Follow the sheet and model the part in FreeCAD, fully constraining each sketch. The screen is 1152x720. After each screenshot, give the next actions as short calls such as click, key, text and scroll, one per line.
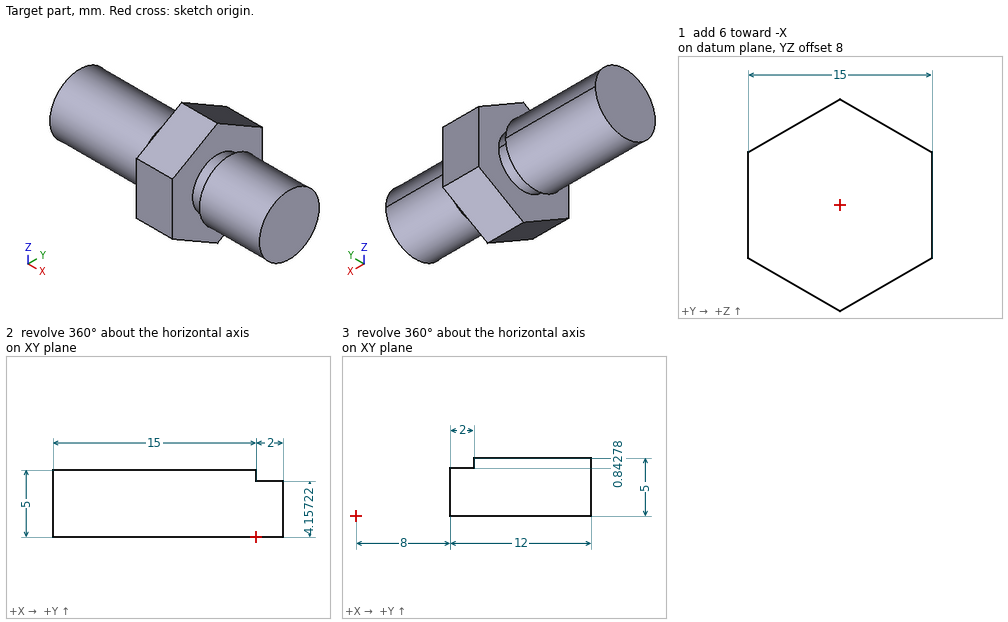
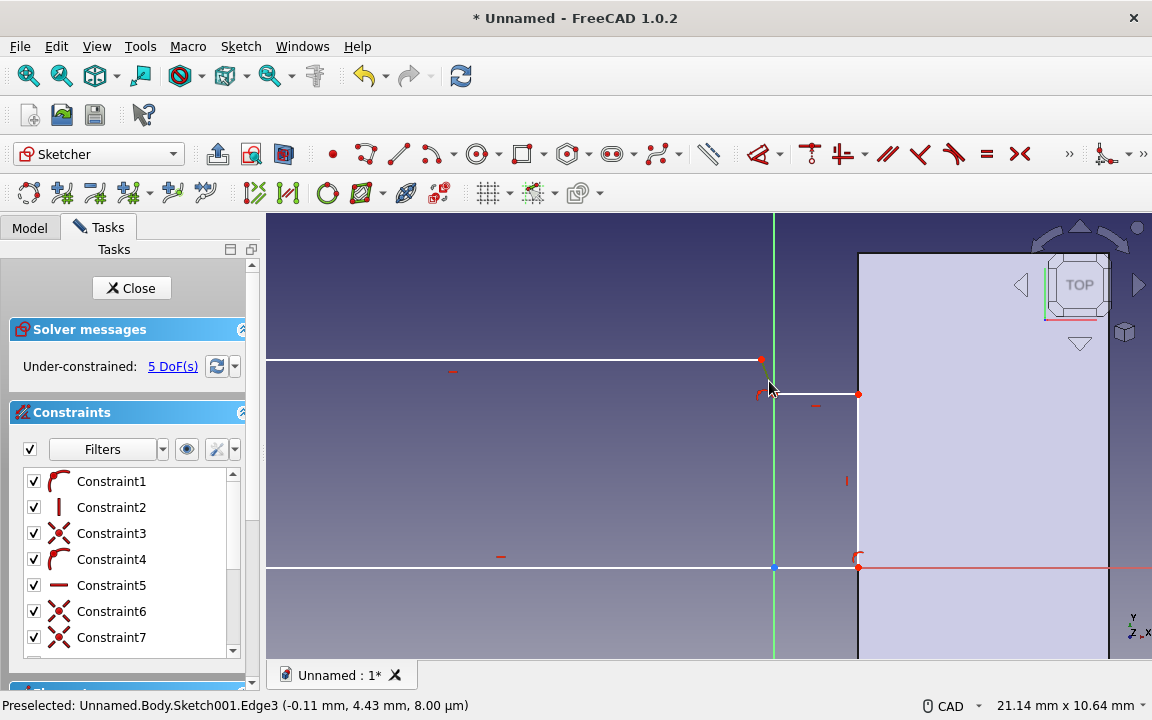
key(v)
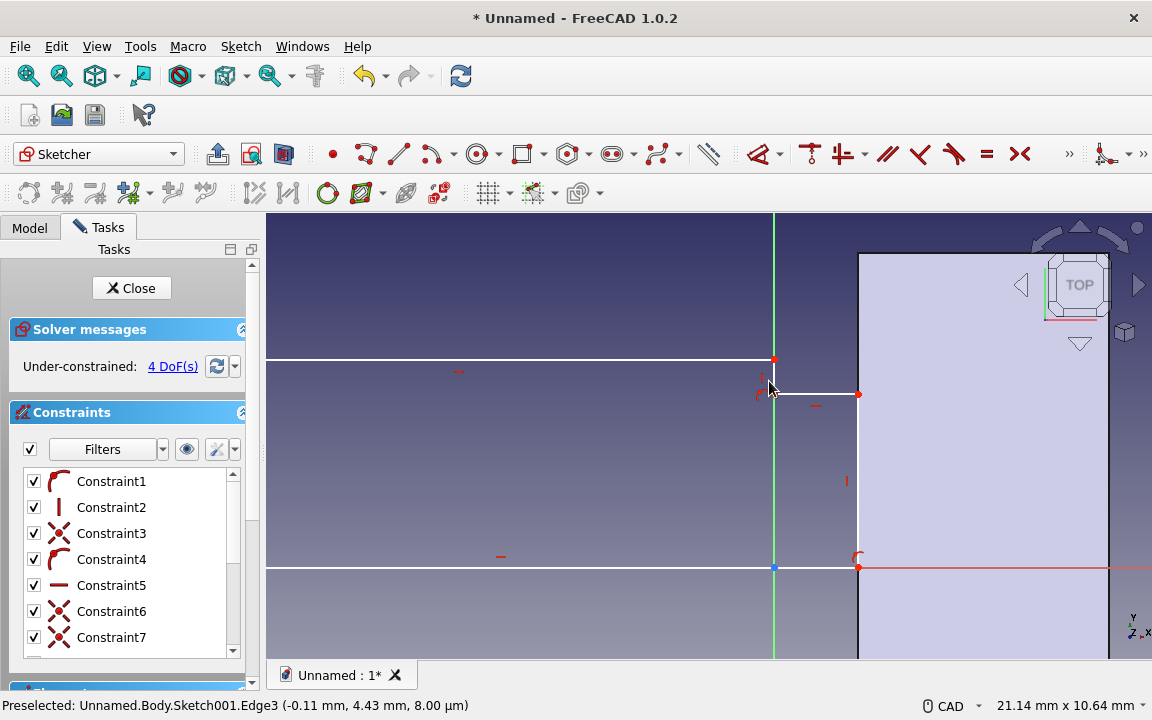
click(833, 394)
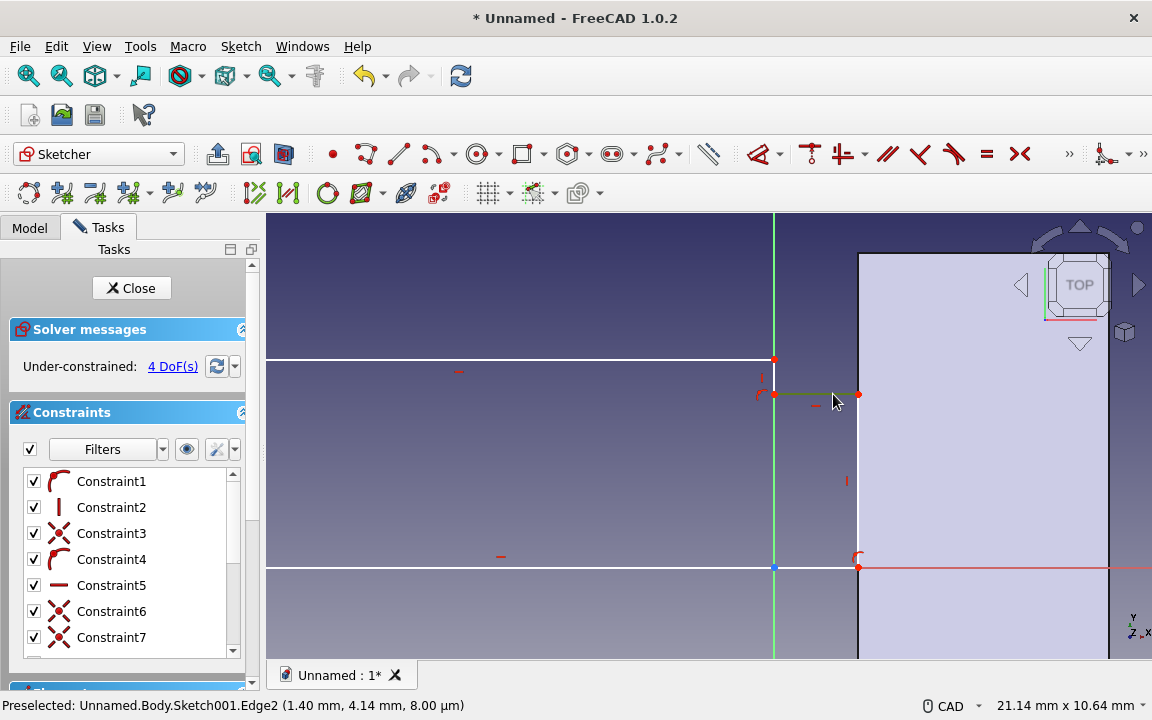
key(l)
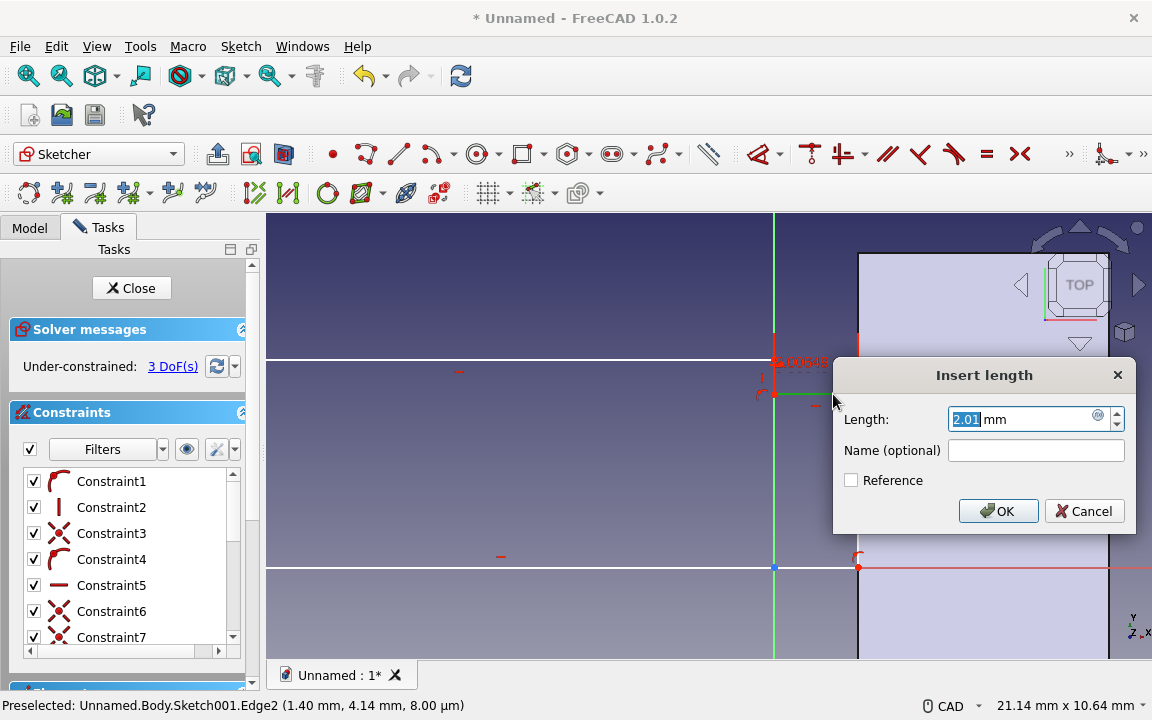
text(2)
key(Return)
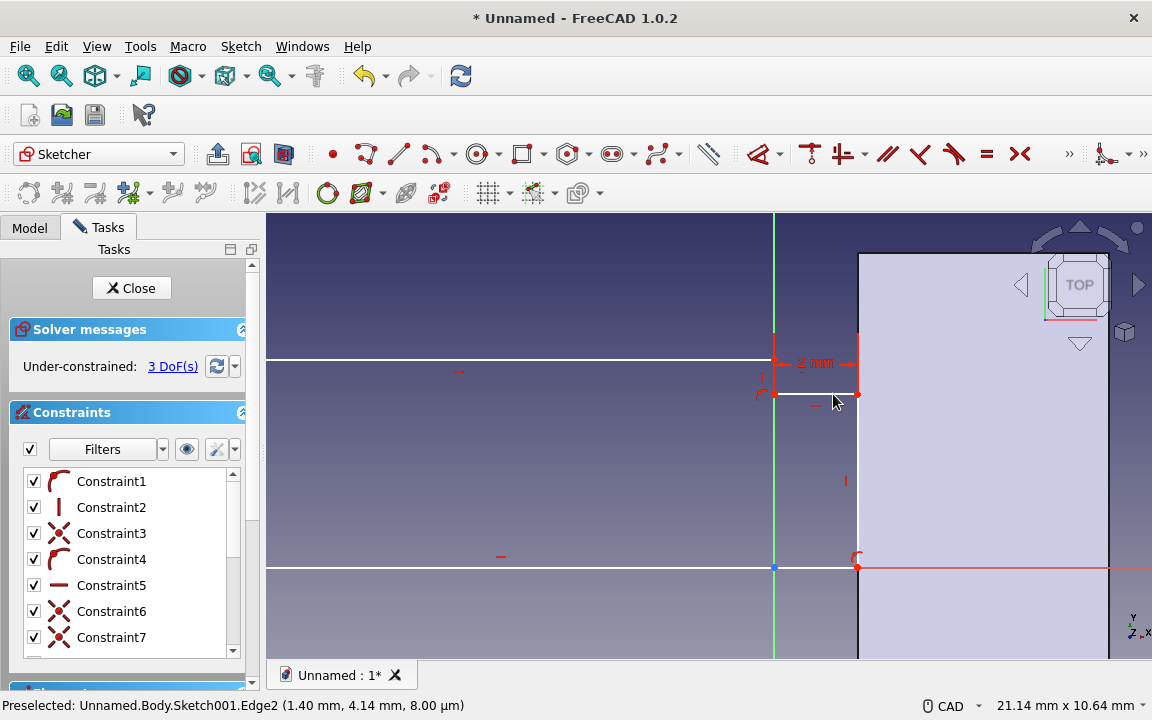
scroll(923, 381, down, 2)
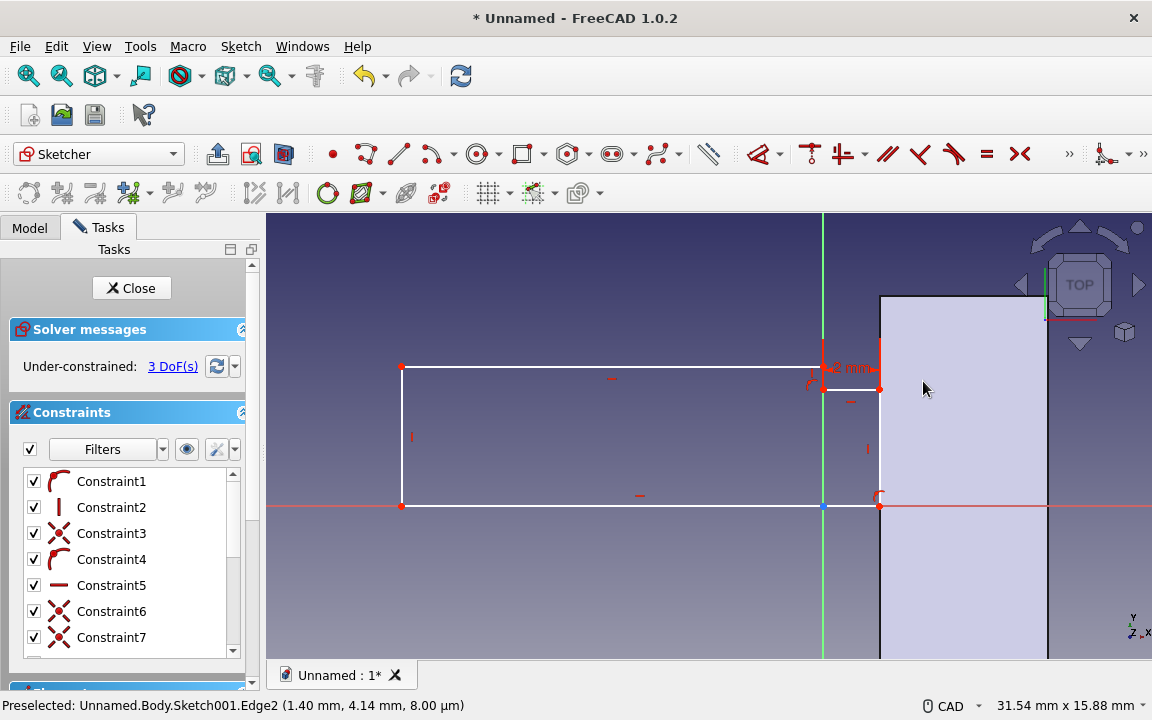
click(402, 409)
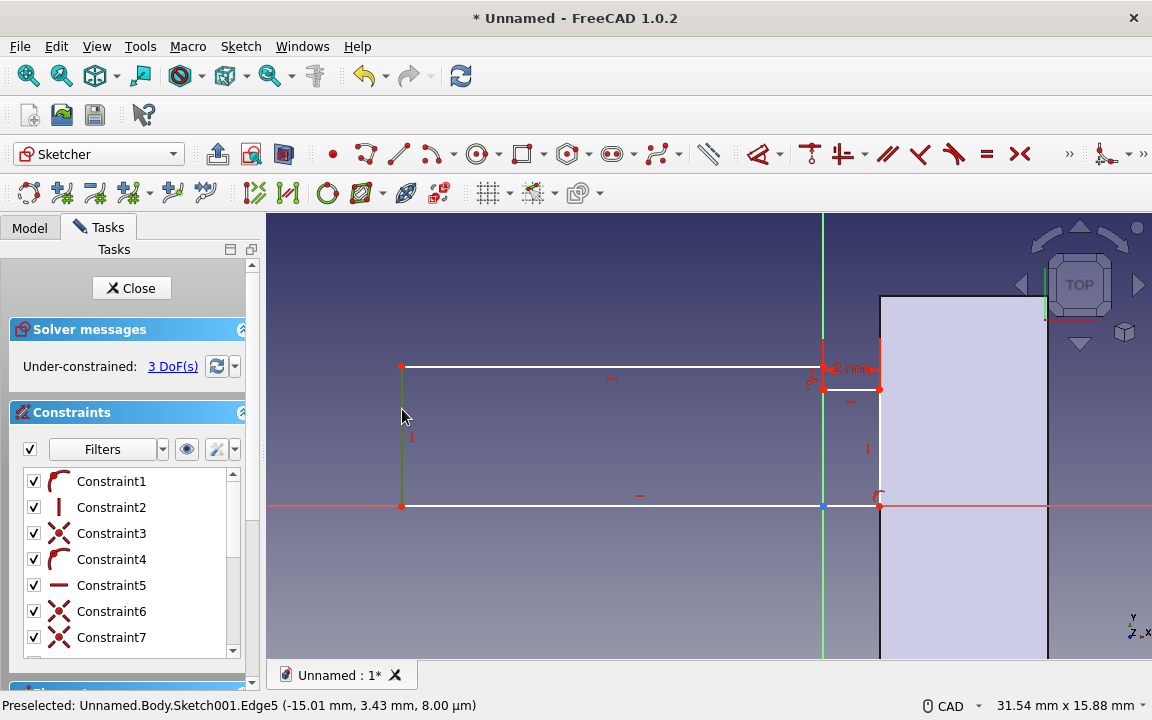
key(i)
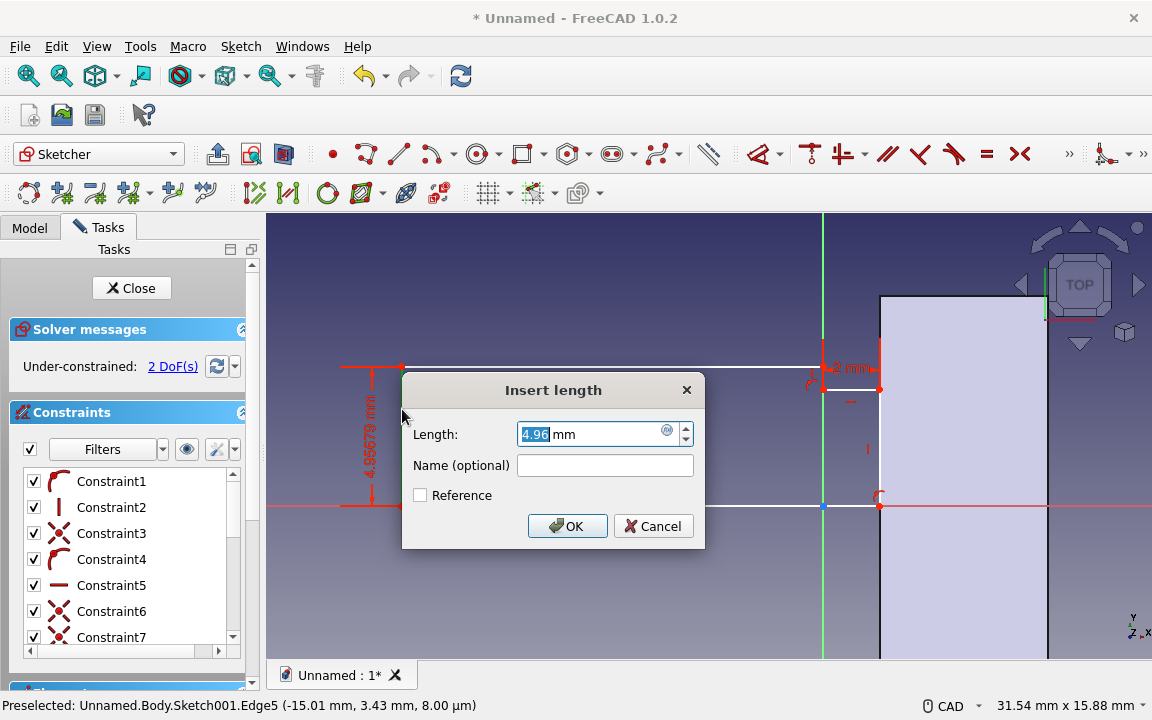
text(5)
key(Return)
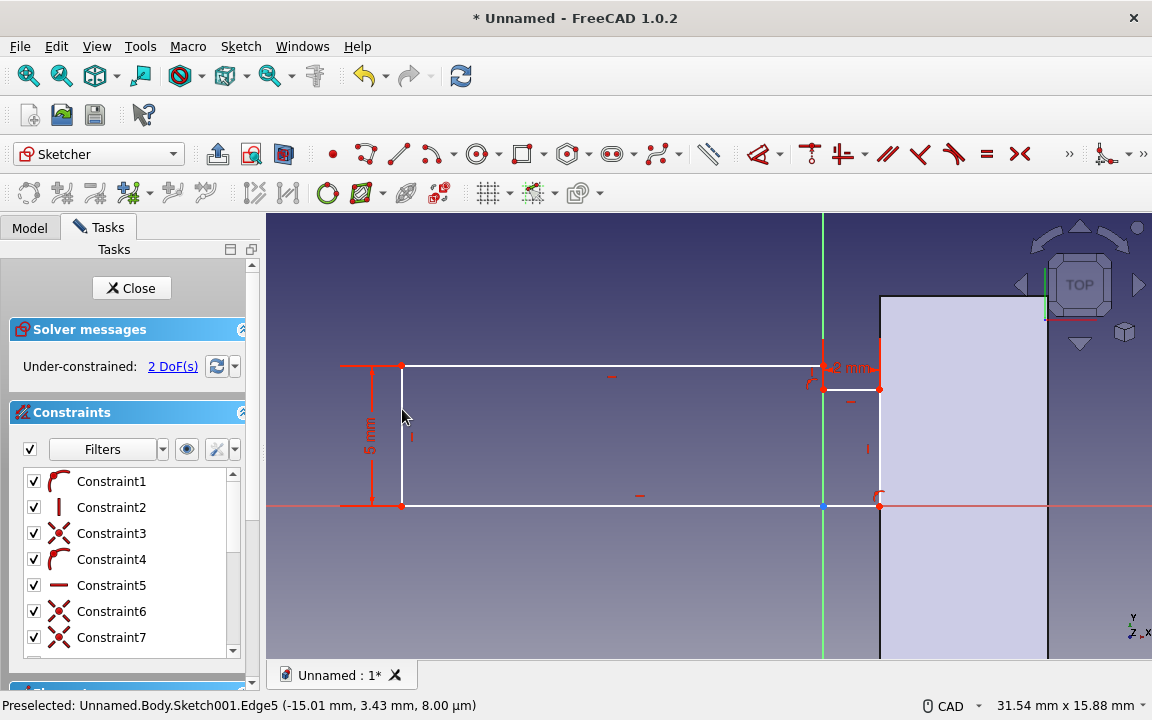
click(697, 366)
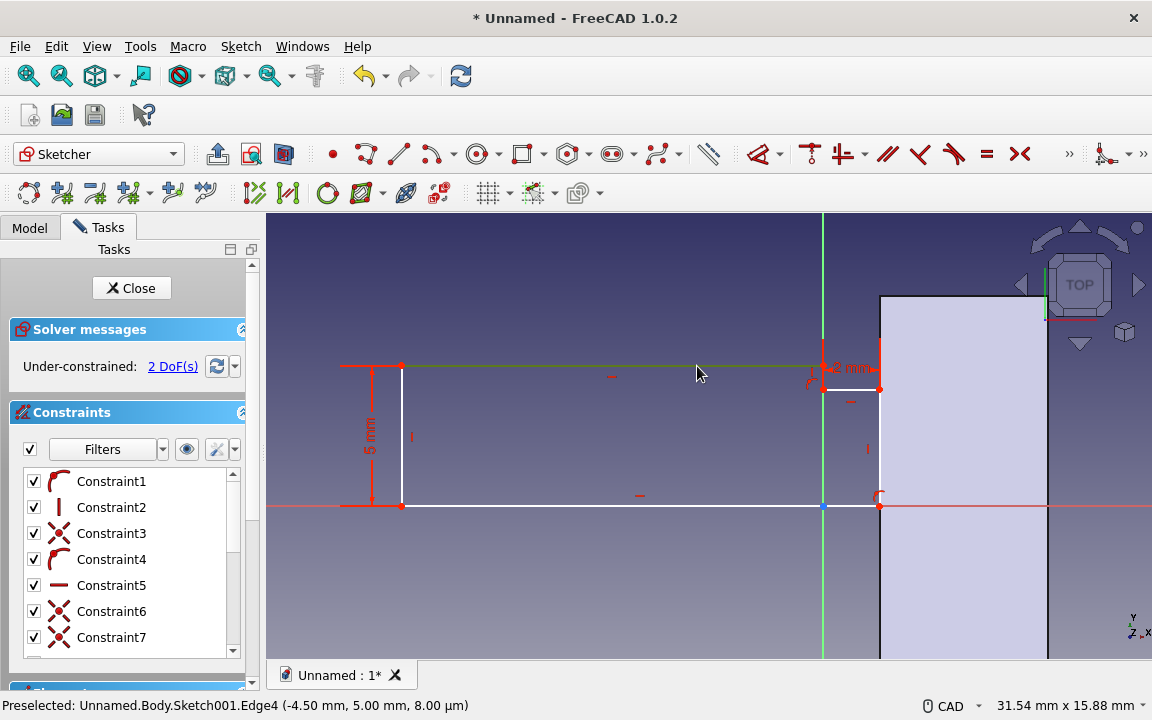
click(780, 154)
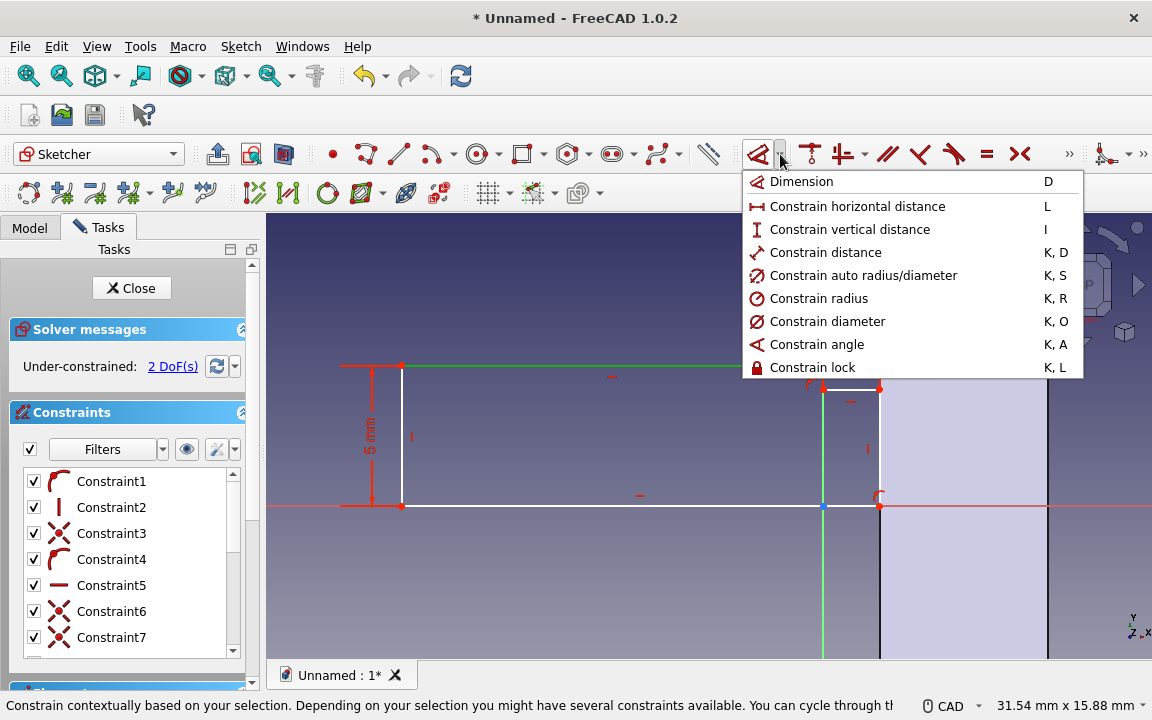
click(913, 206)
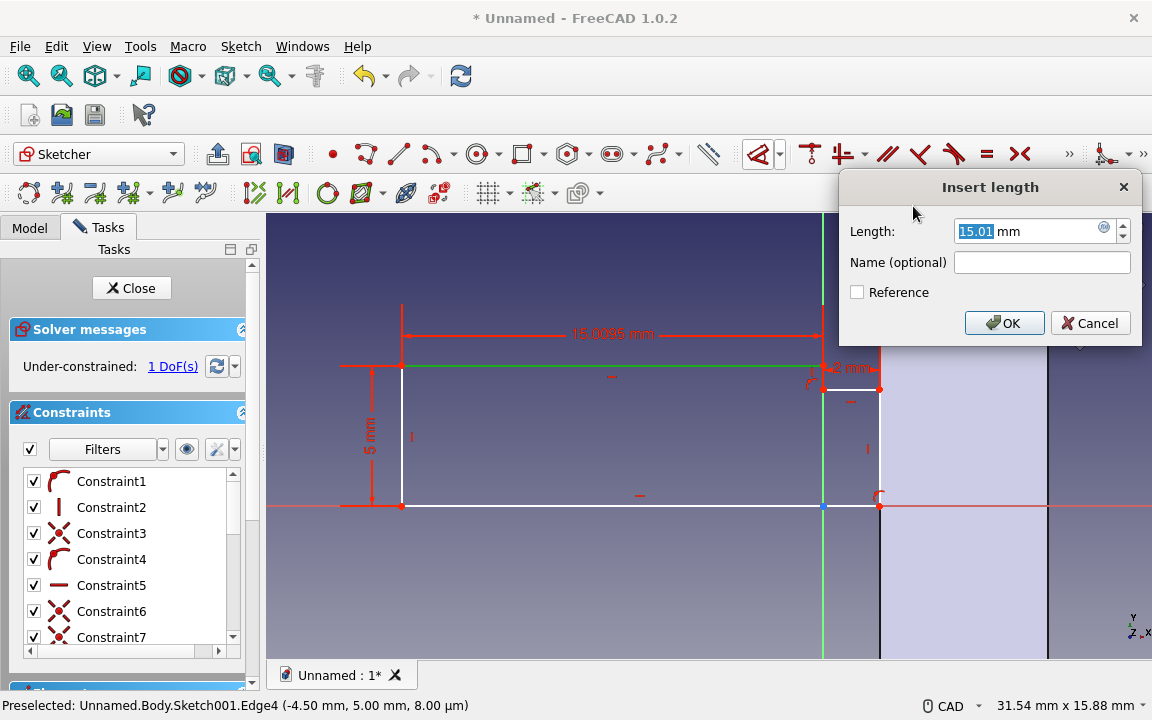
text(15)
key(Return)